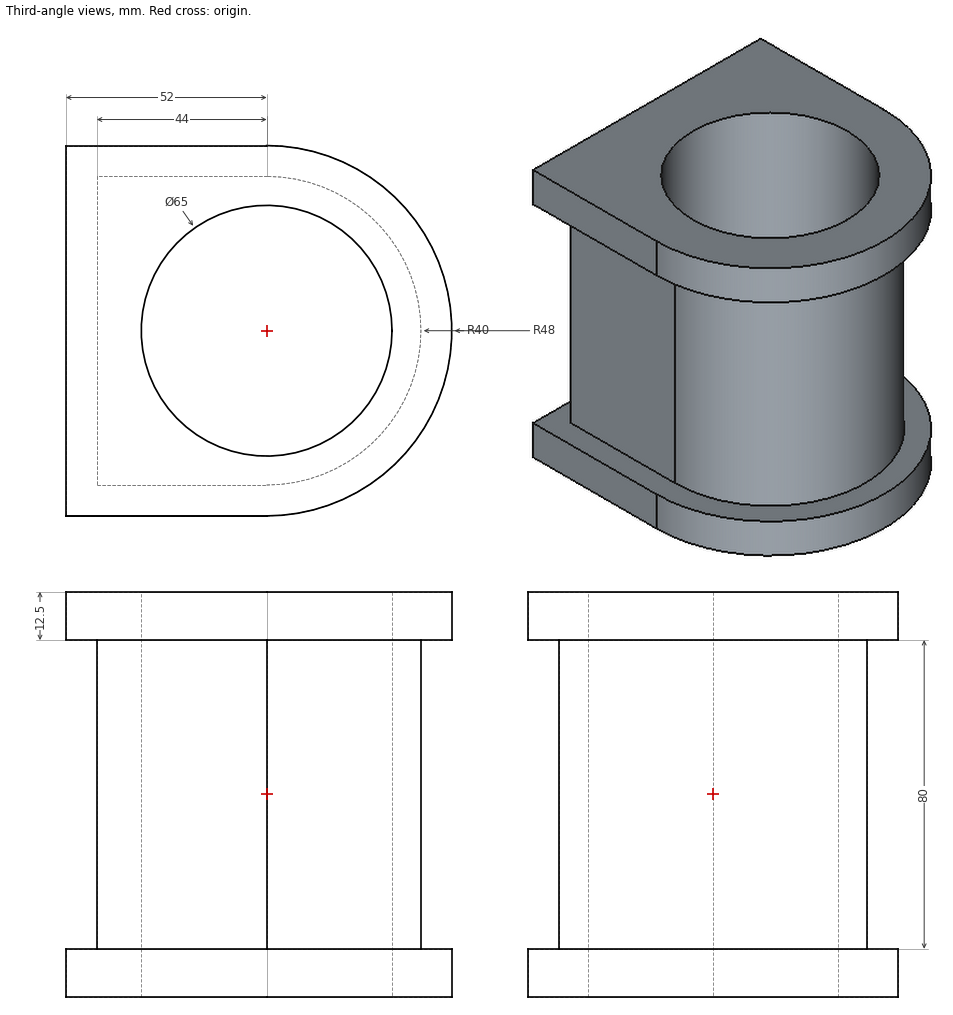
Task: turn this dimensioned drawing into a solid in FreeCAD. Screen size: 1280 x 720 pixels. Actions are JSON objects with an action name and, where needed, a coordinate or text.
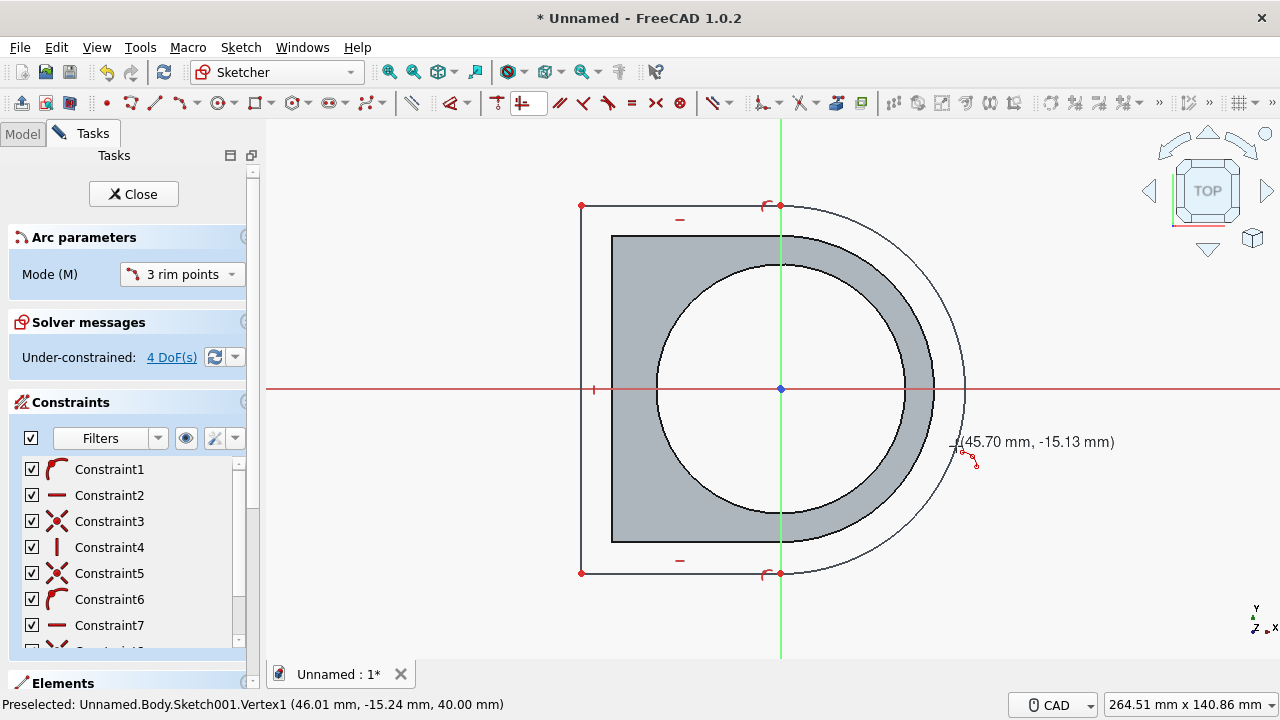
{"action": "left_click", "coordinate": [218, 104]}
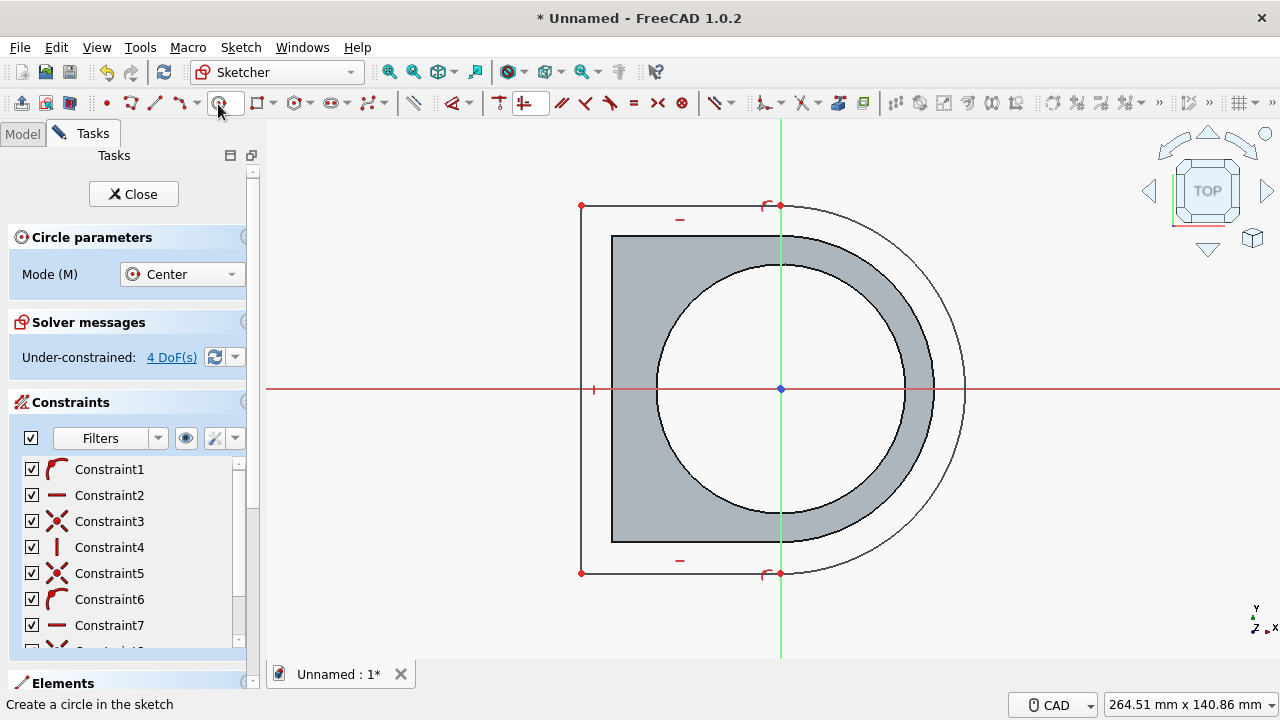
{"action": "left_click", "coordinate": [781, 389]}
{"action": "left_click", "coordinate": [869, 301]}
{"action": "key", "text": "Escape"}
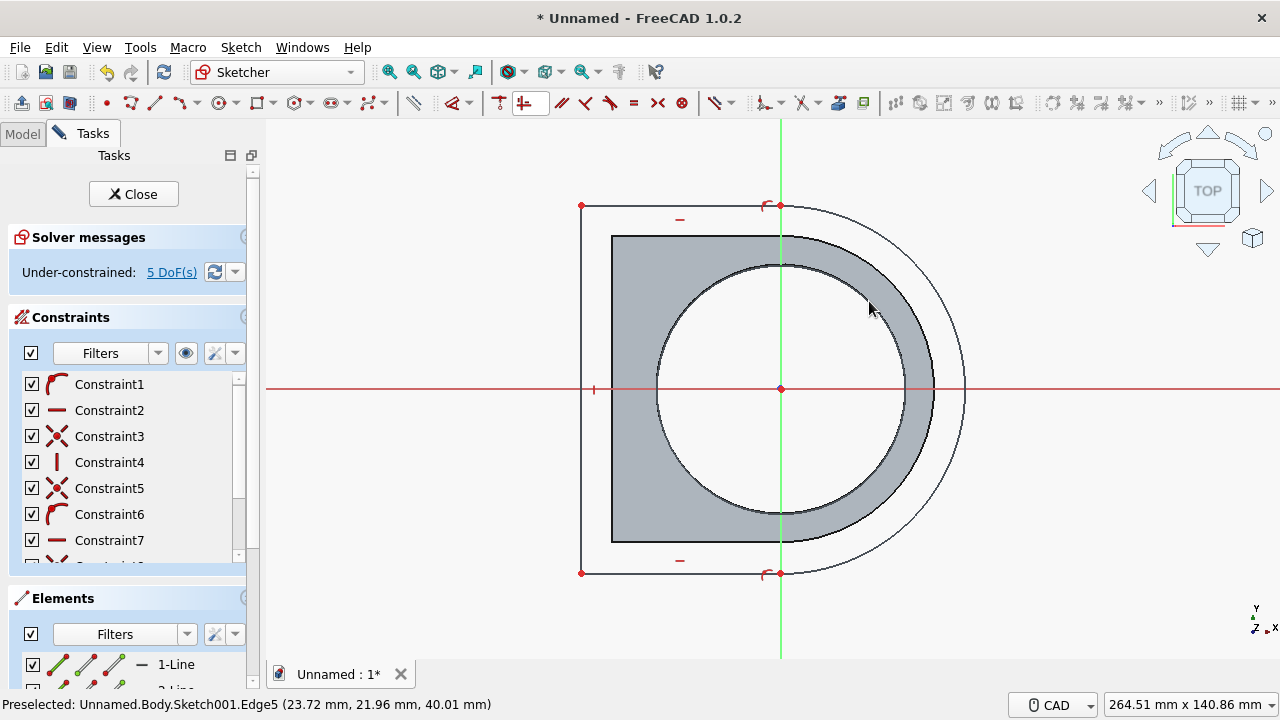
{"action": "left_click_drag", "start_coordinate": [771, 379], "coordinate": [791, 400]}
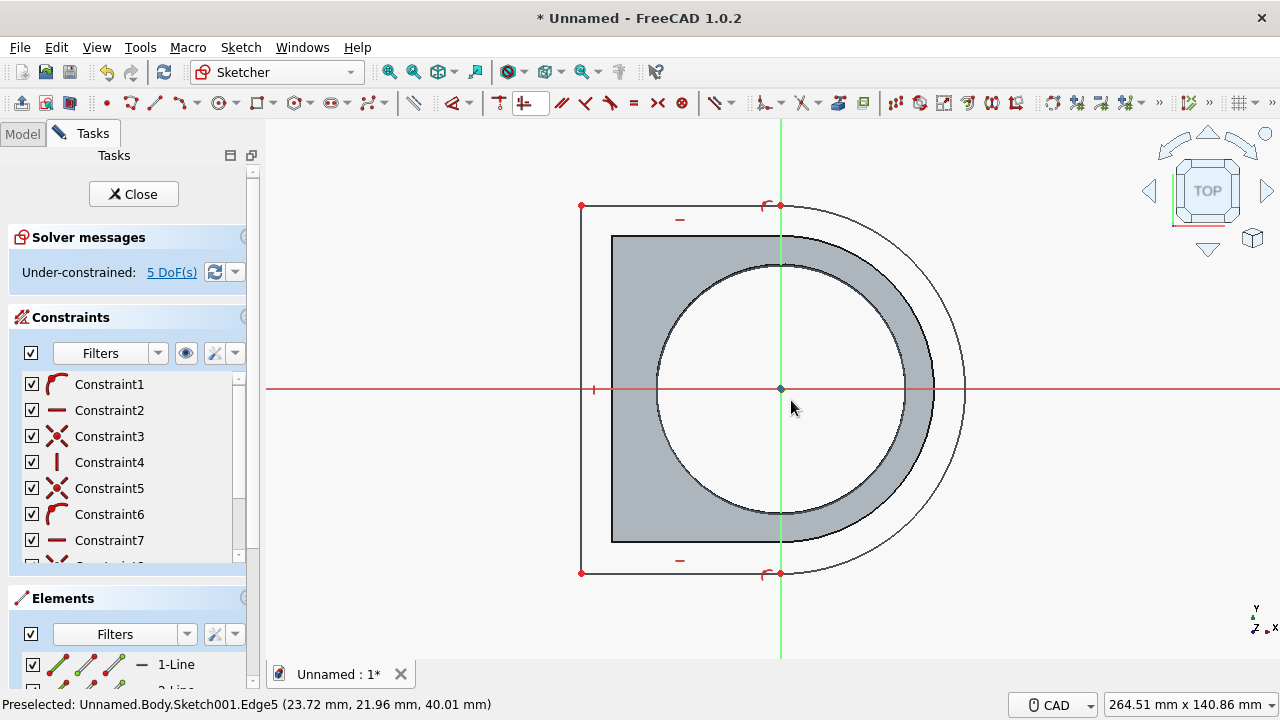
{"action": "left_click", "coordinate": [500, 104]}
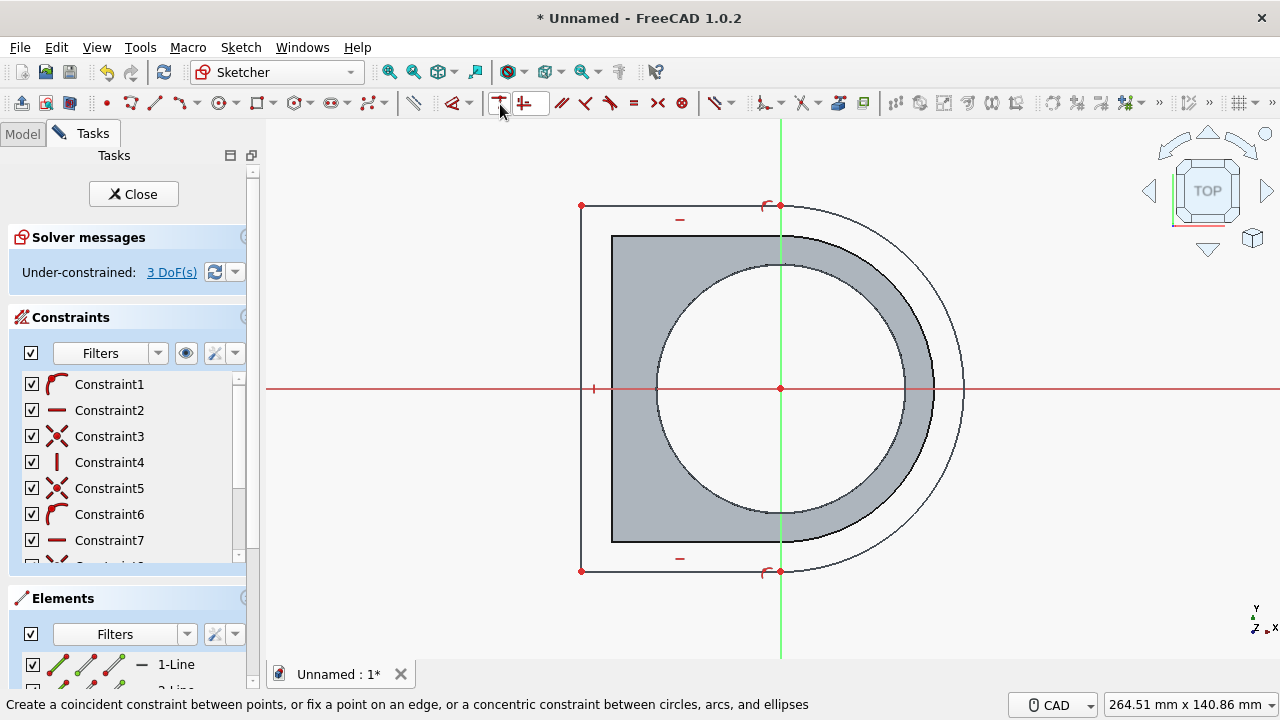
{"action": "left_click", "coordinate": [929, 497]}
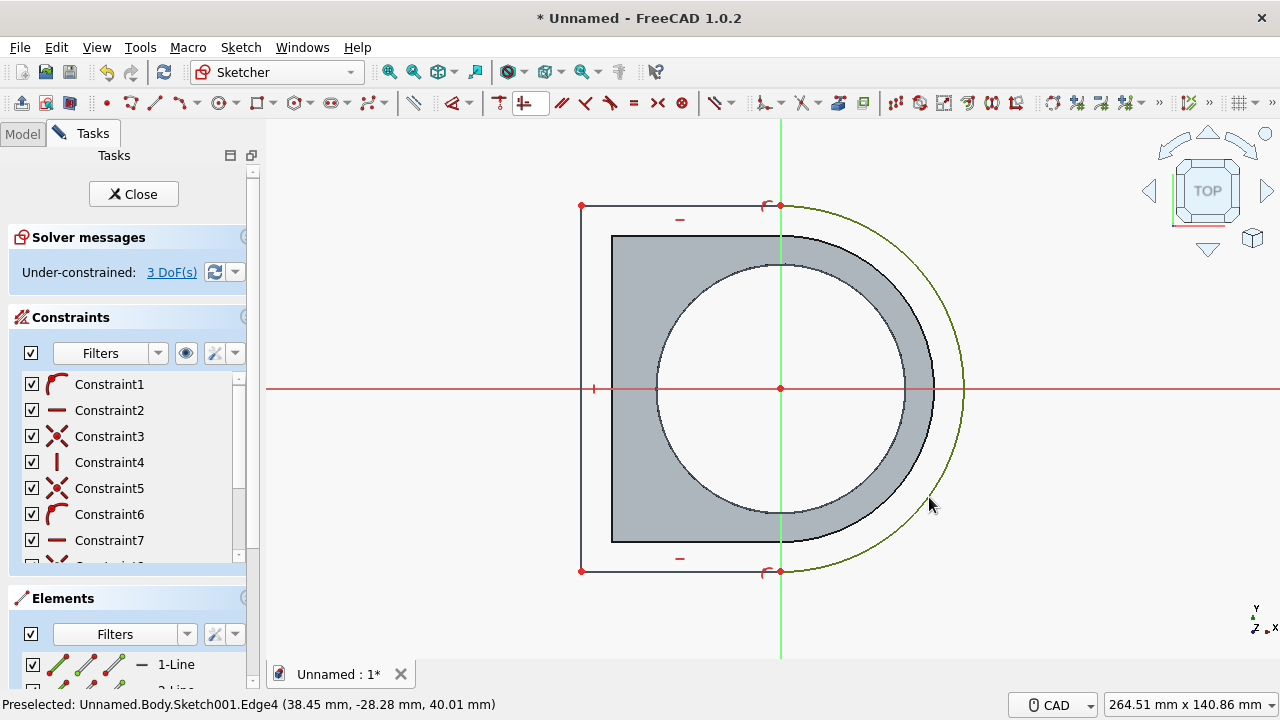
{"action": "key", "text": "k r"}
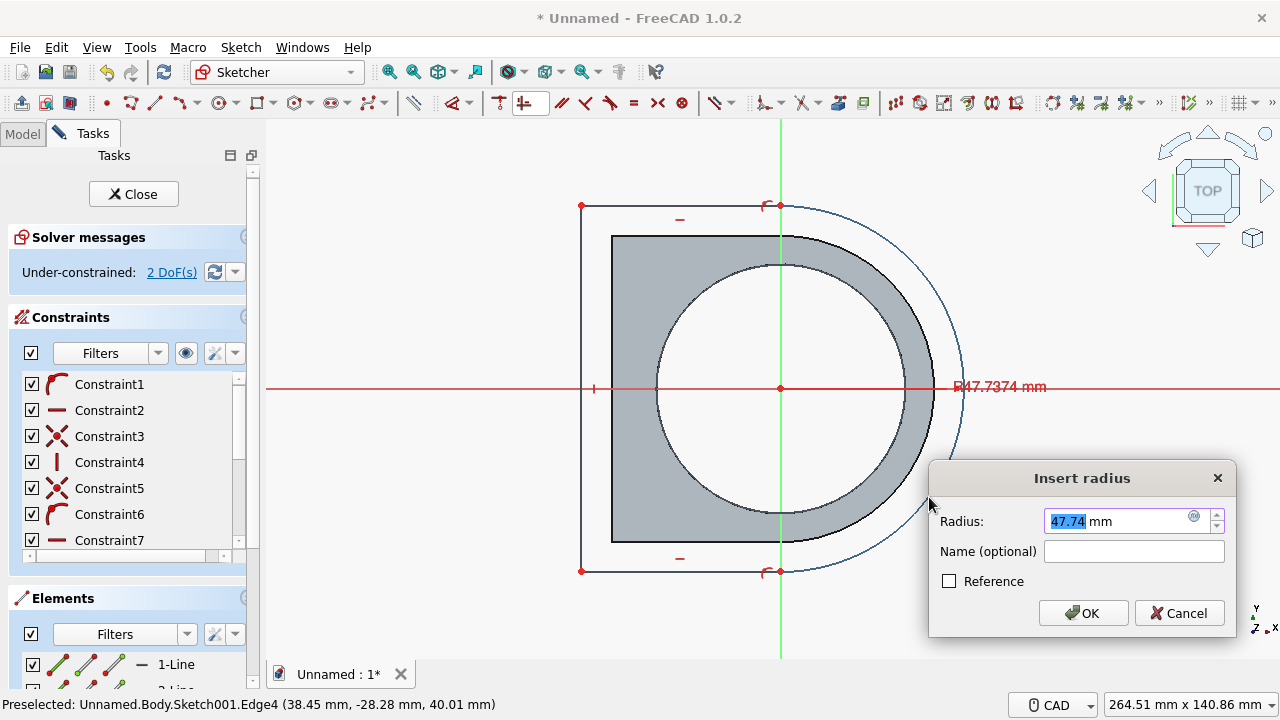
{"action": "type", "text": "48"}
{"action": "key", "text": "Return"}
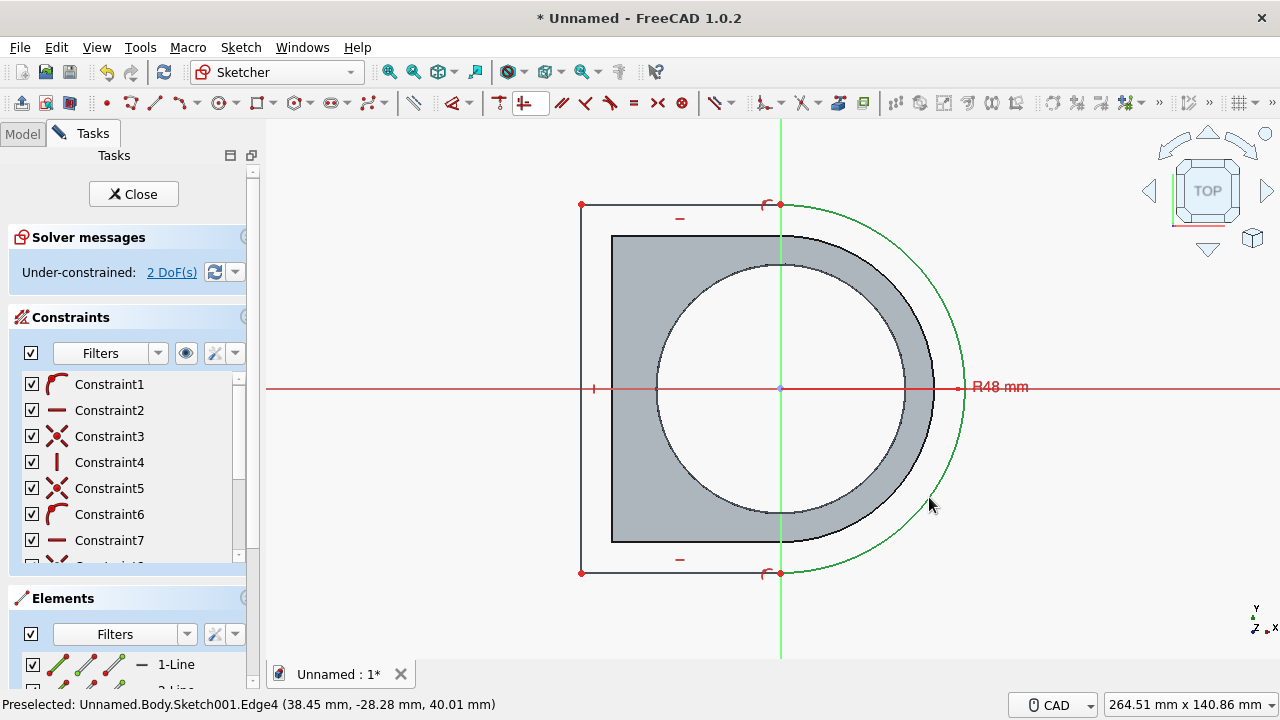
{"action": "left_click", "coordinate": [869, 301]}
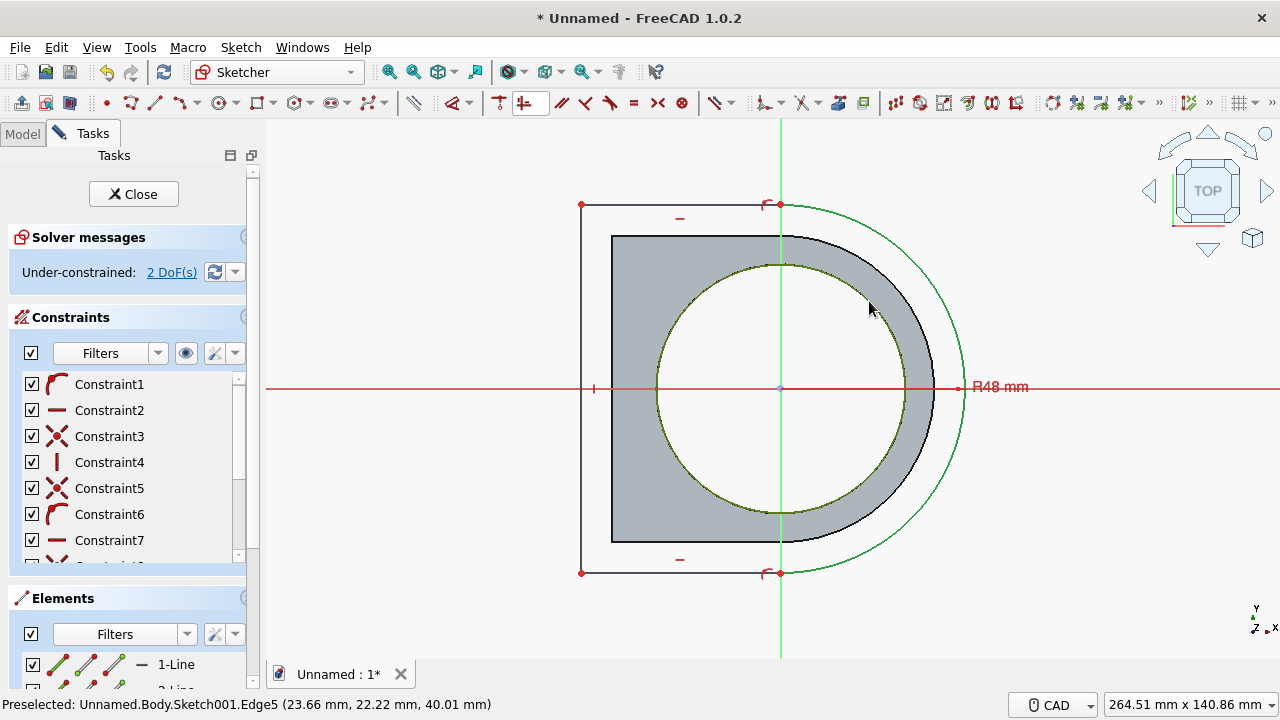
{"action": "left_click", "coordinate": [472, 104]}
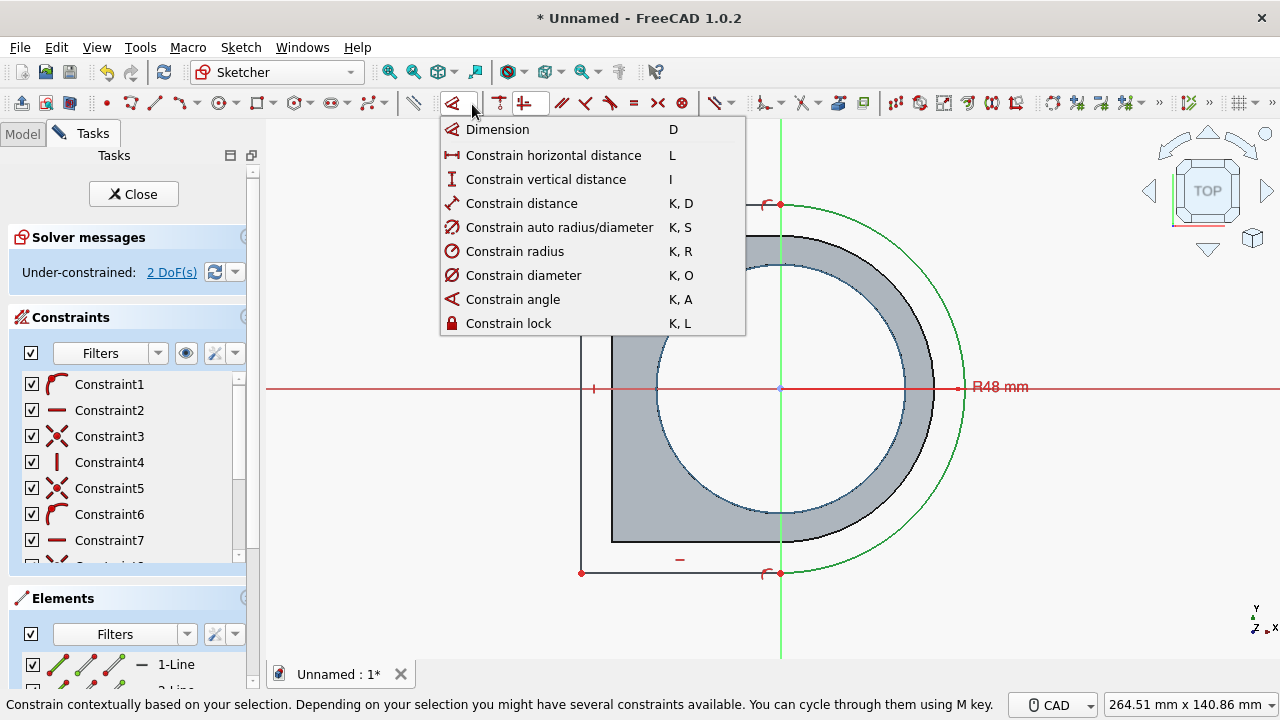
{"action": "left_click", "coordinate": [593, 275]}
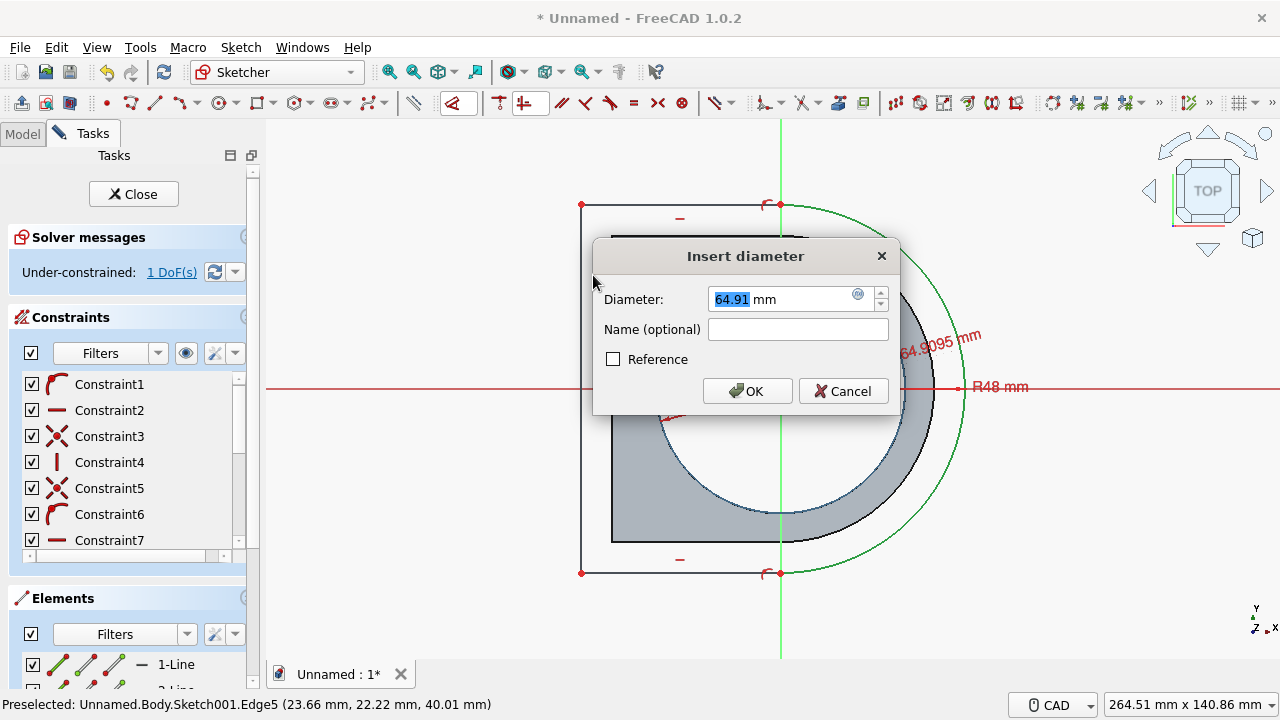
{"action": "type", "text": "65"}
{"action": "key", "text": "Return"}